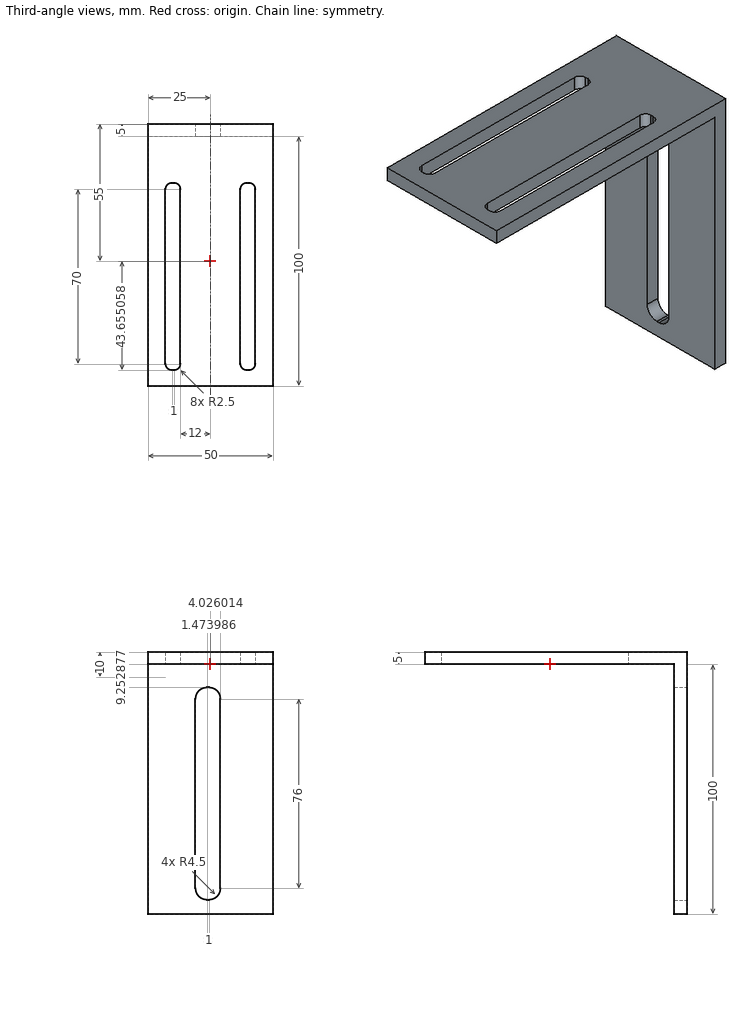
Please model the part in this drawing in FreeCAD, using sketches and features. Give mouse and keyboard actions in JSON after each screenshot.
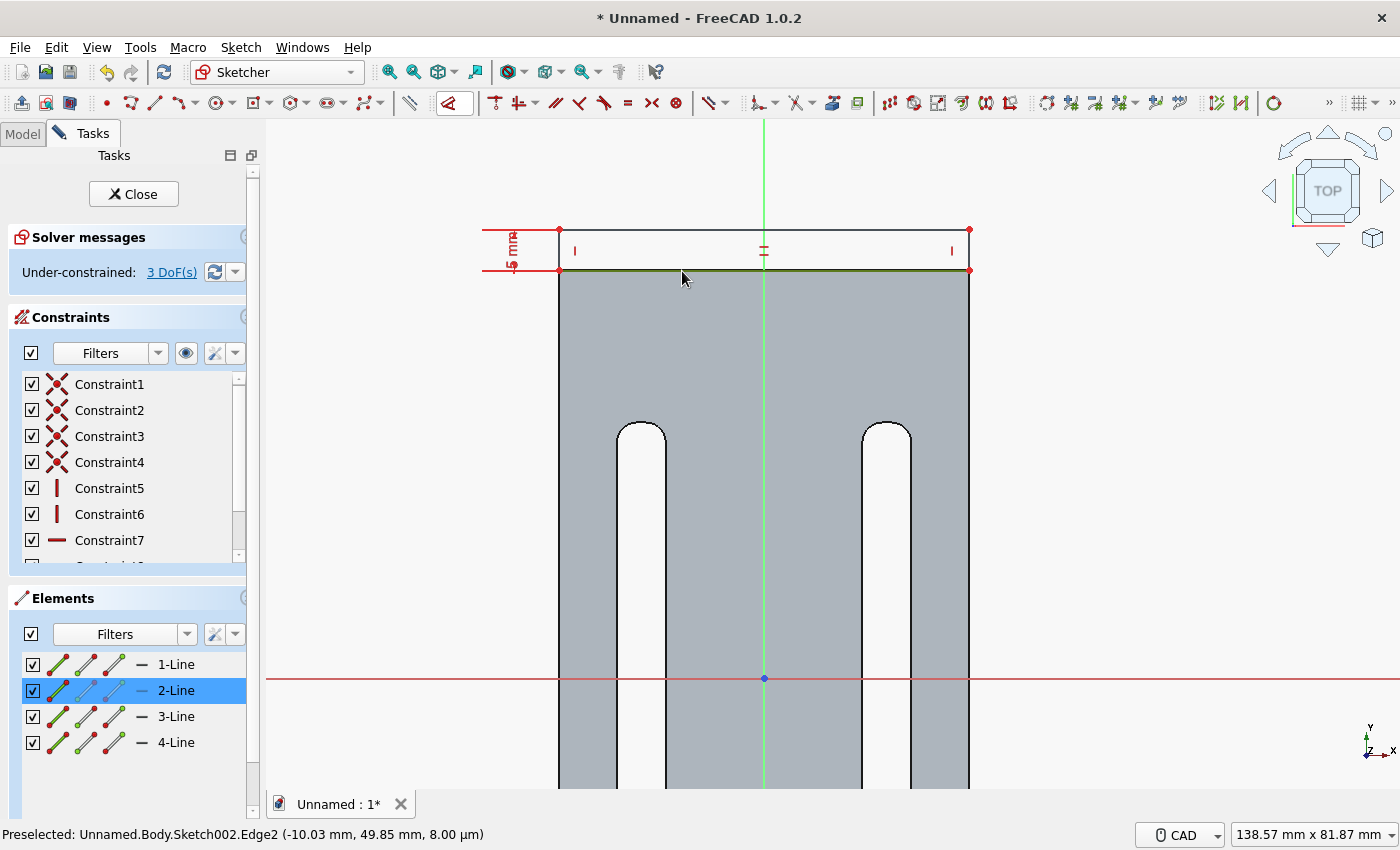
{"action": "key", "text": "l"}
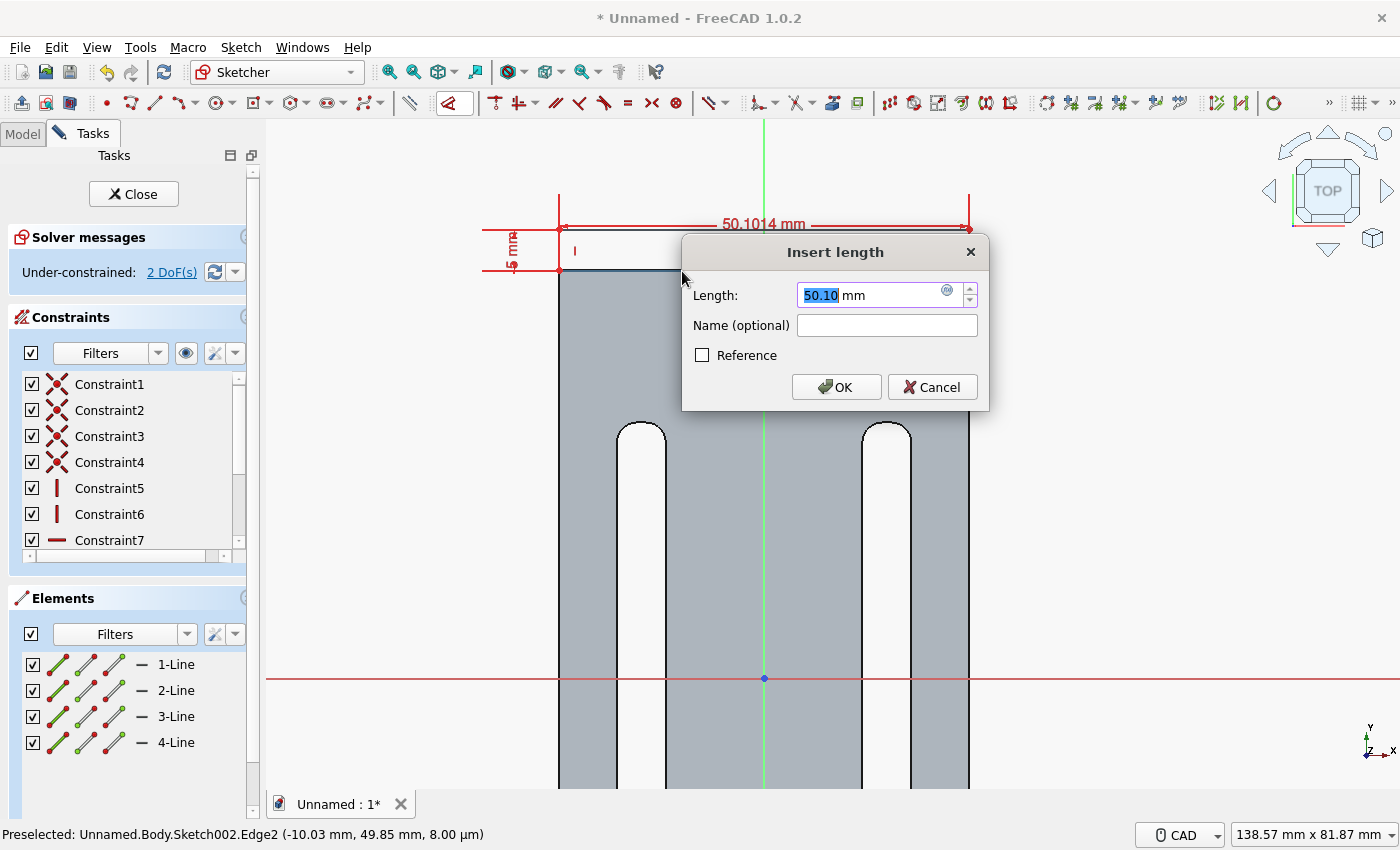
{"action": "type", "text": "50"}
{"action": "key", "text": "Return"}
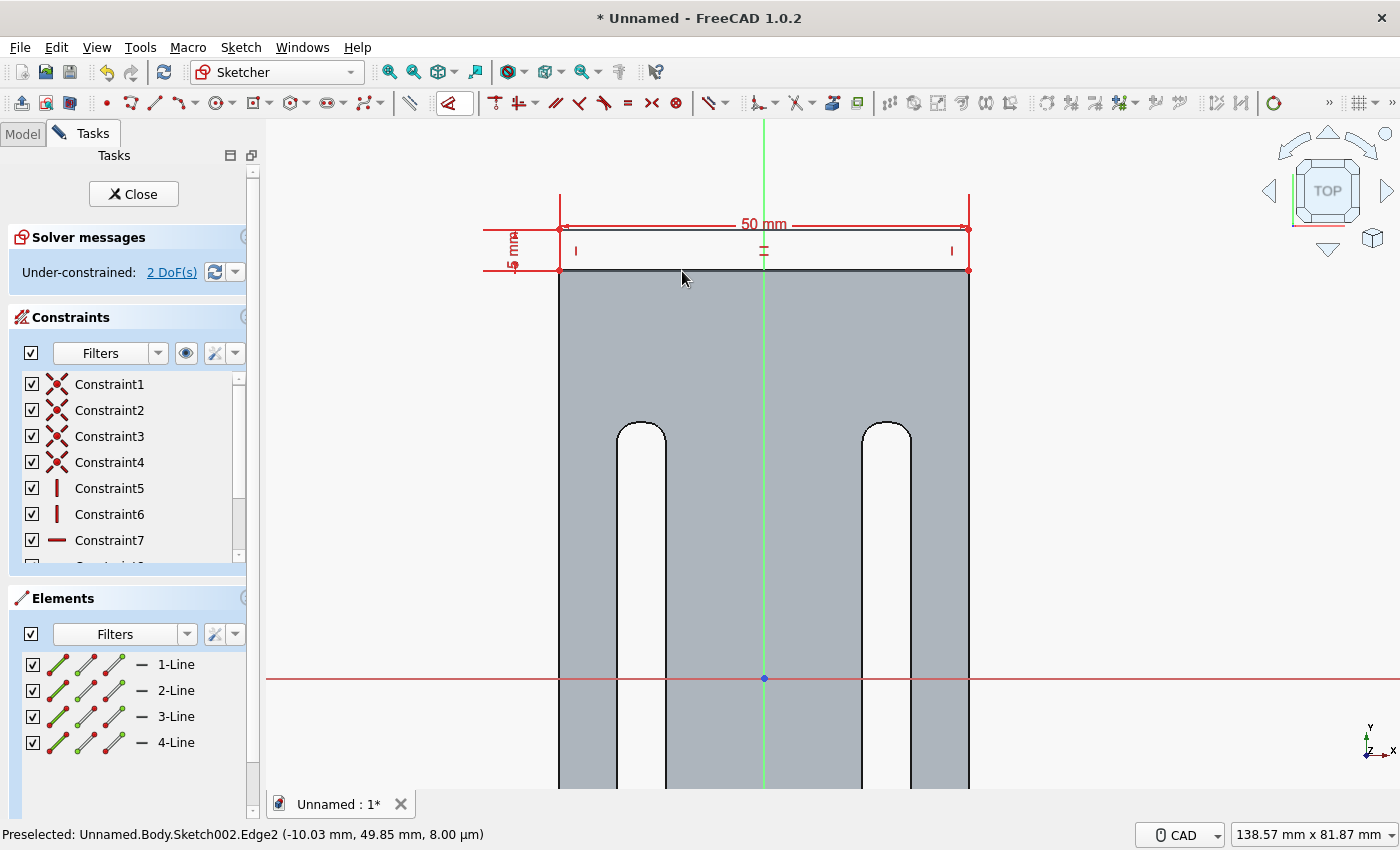
{"action": "left_click", "coordinate": [560, 230]}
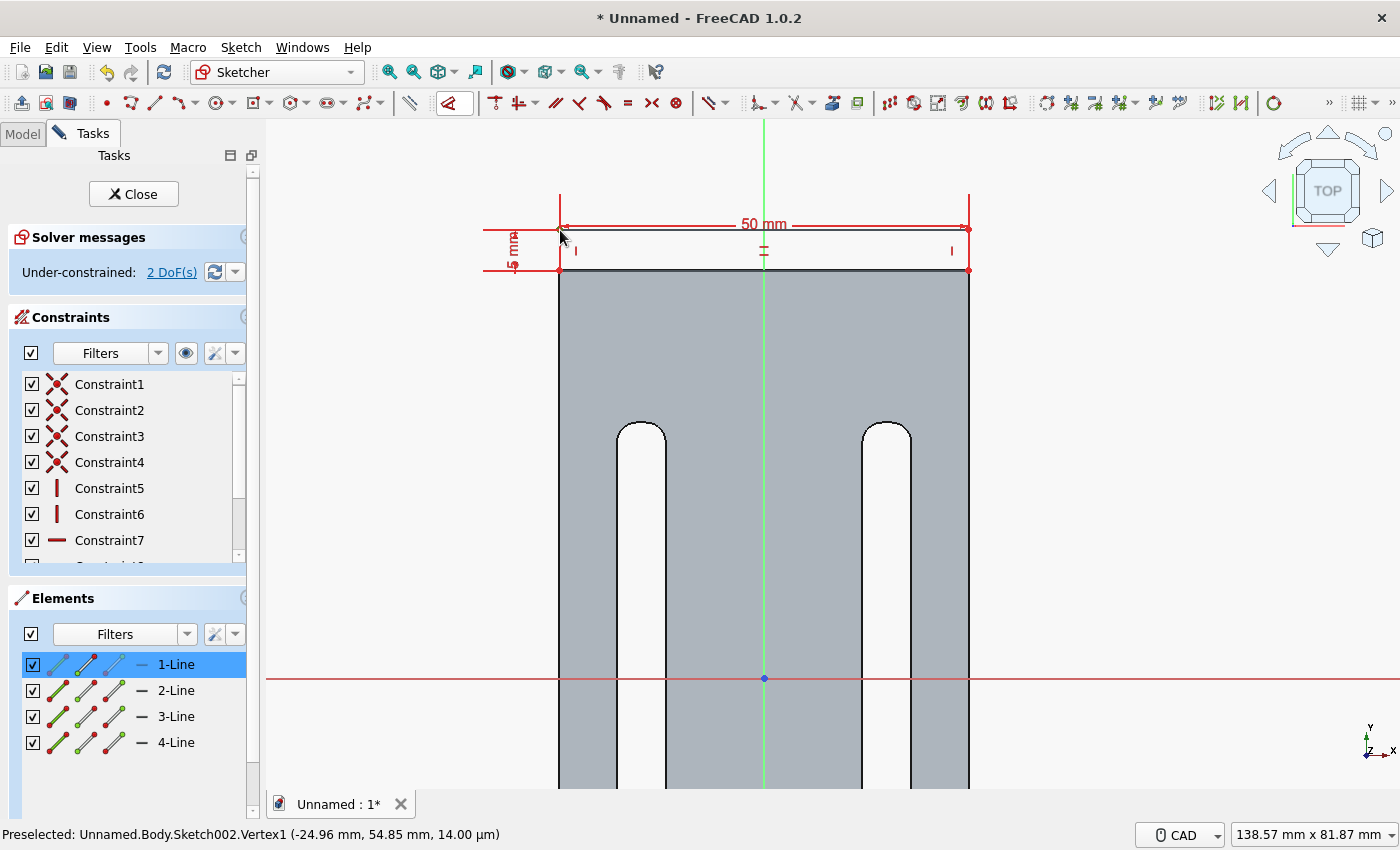
{"action": "left_click", "coordinate": [468, 104]}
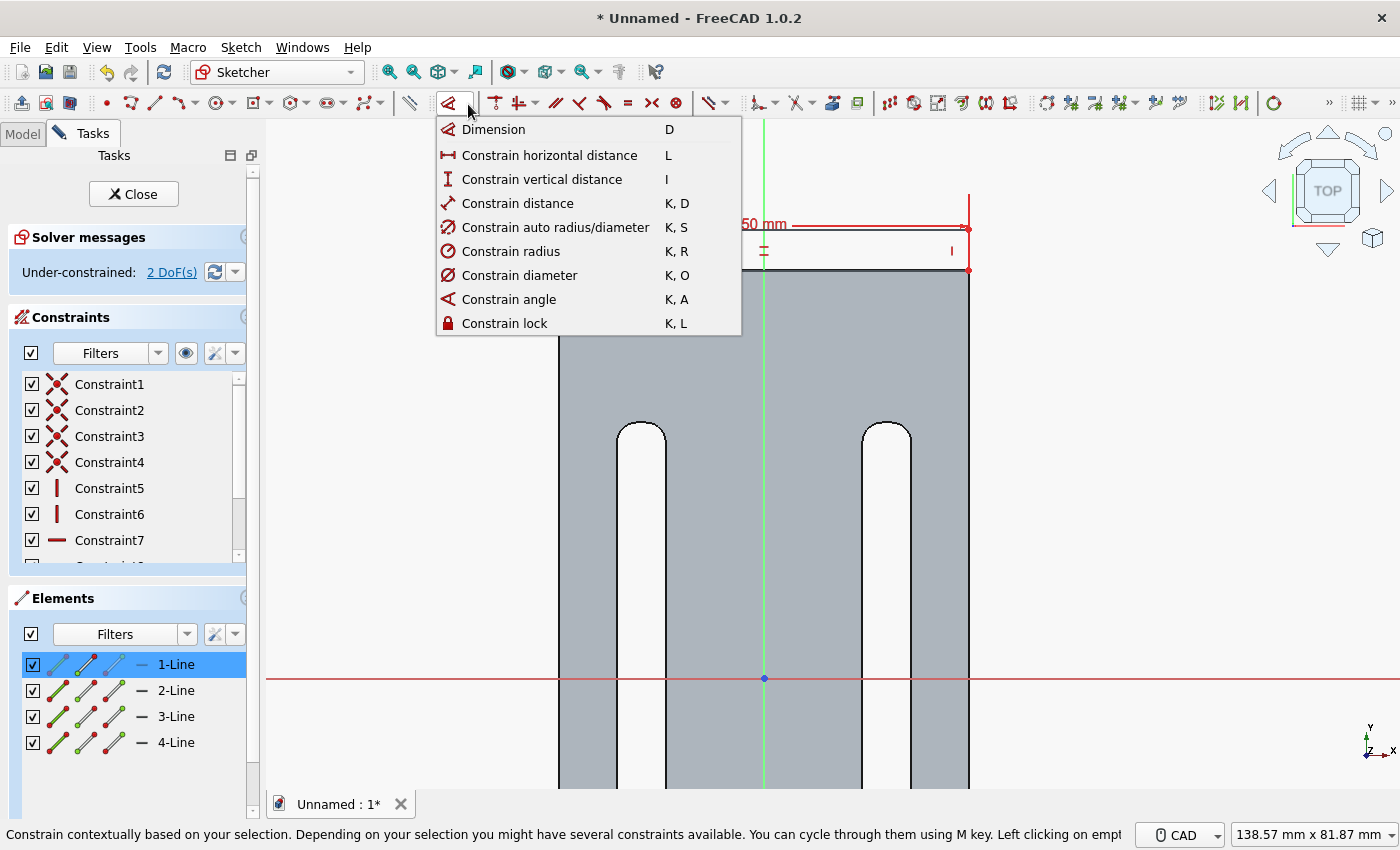
{"action": "left_click", "coordinate": [589, 155]}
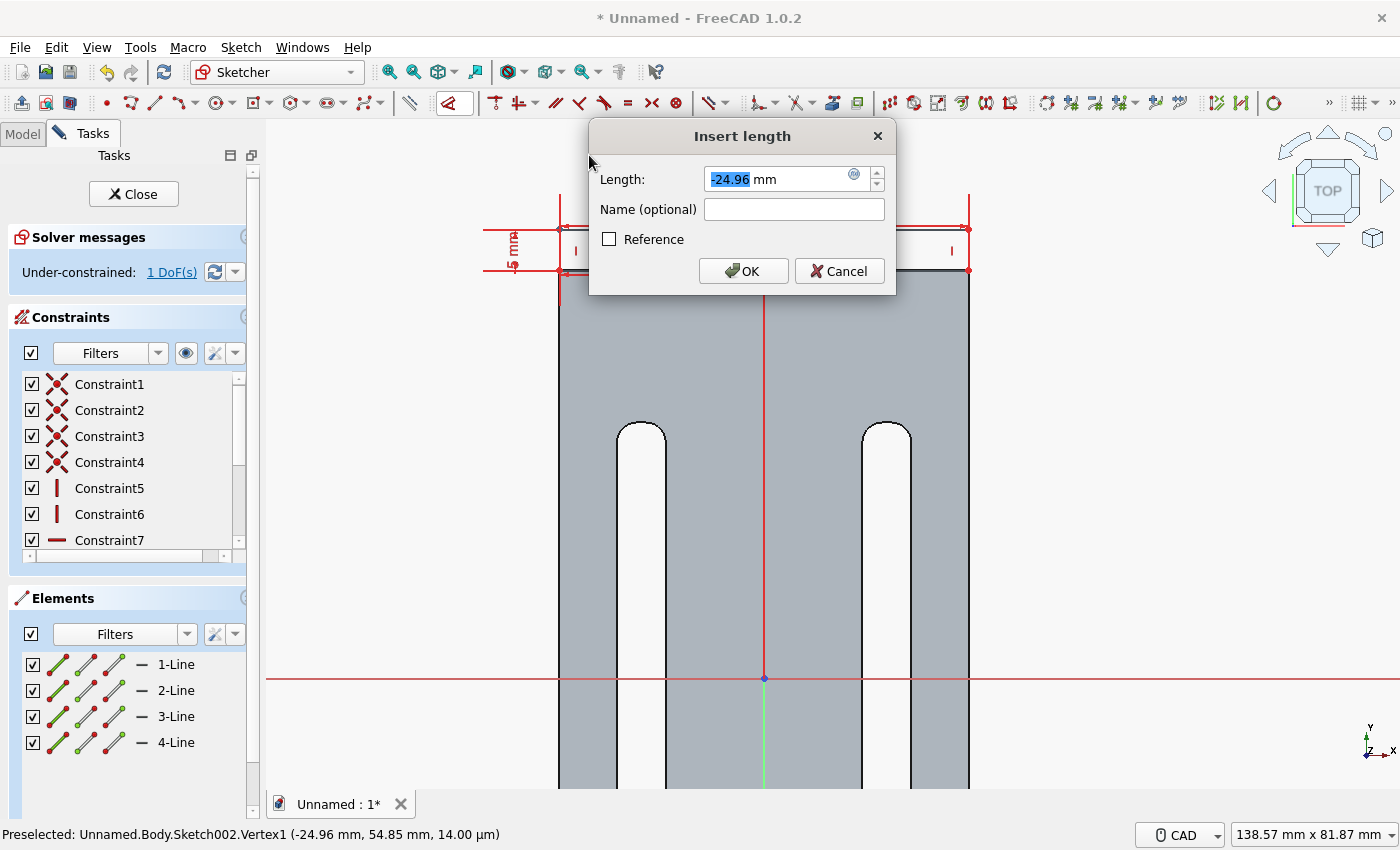
{"action": "type", "text": "-25"}
{"action": "key", "text": "Return"}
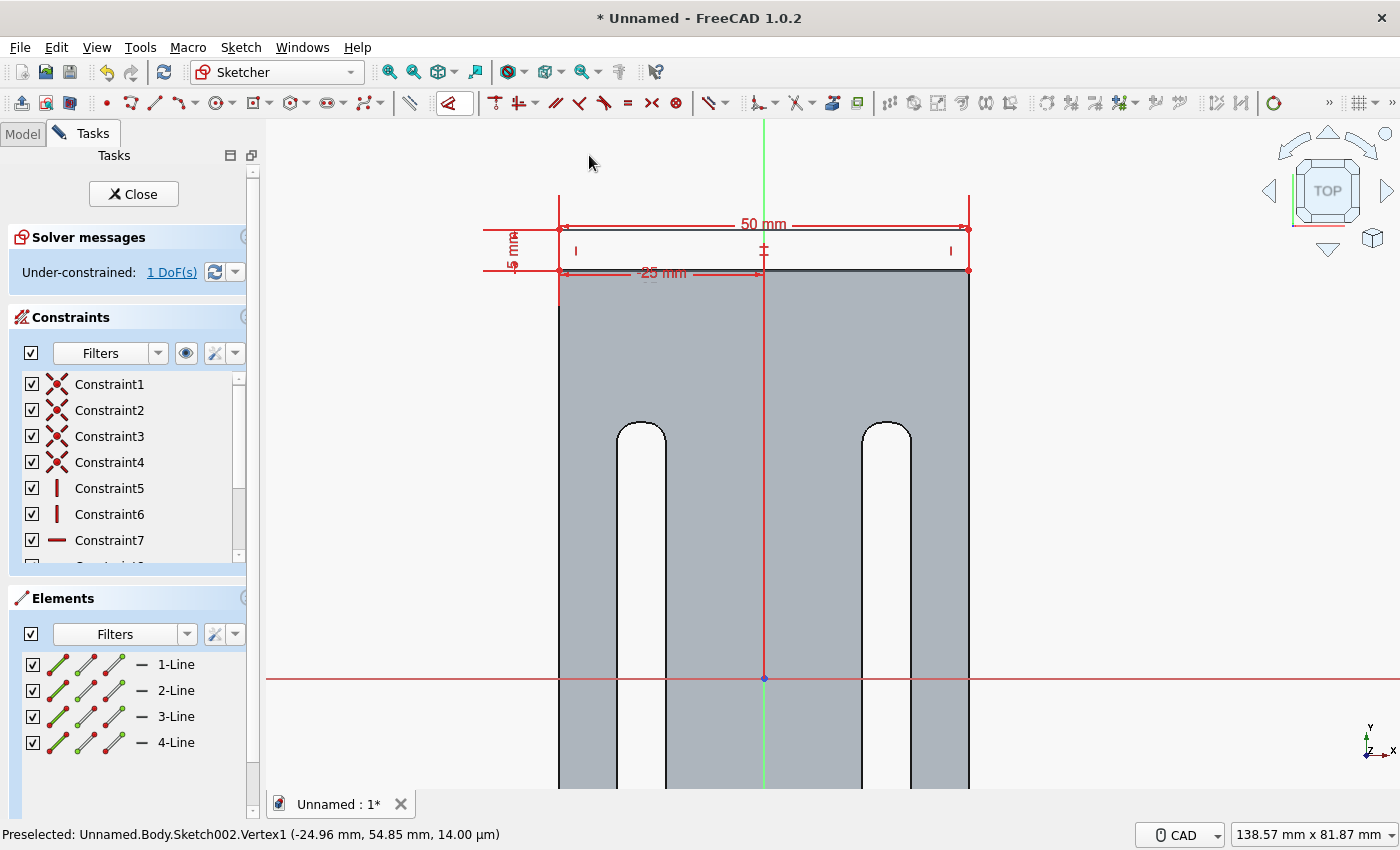
{"action": "left_click", "coordinate": [559, 230]}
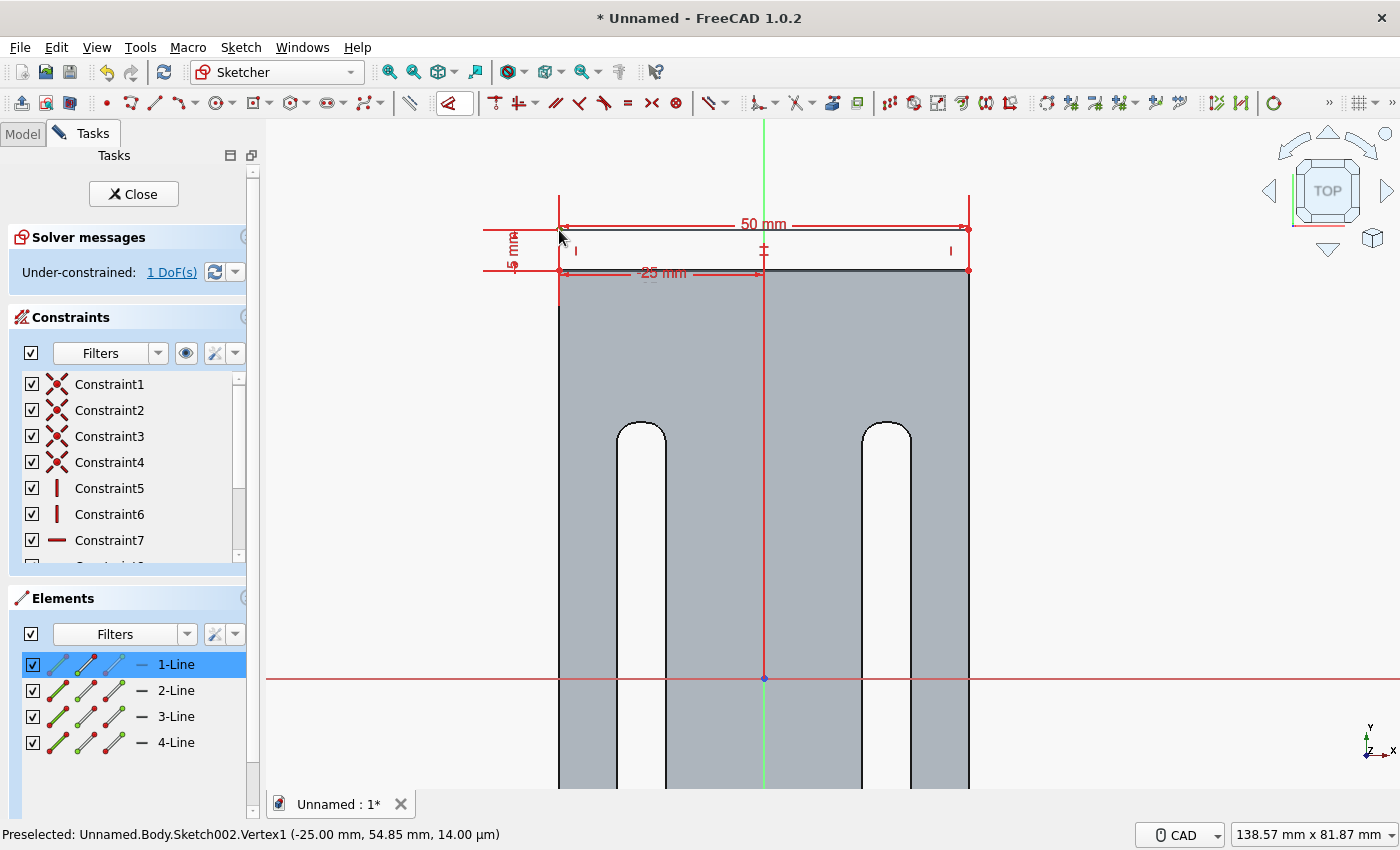
{"action": "key", "text": "i"}